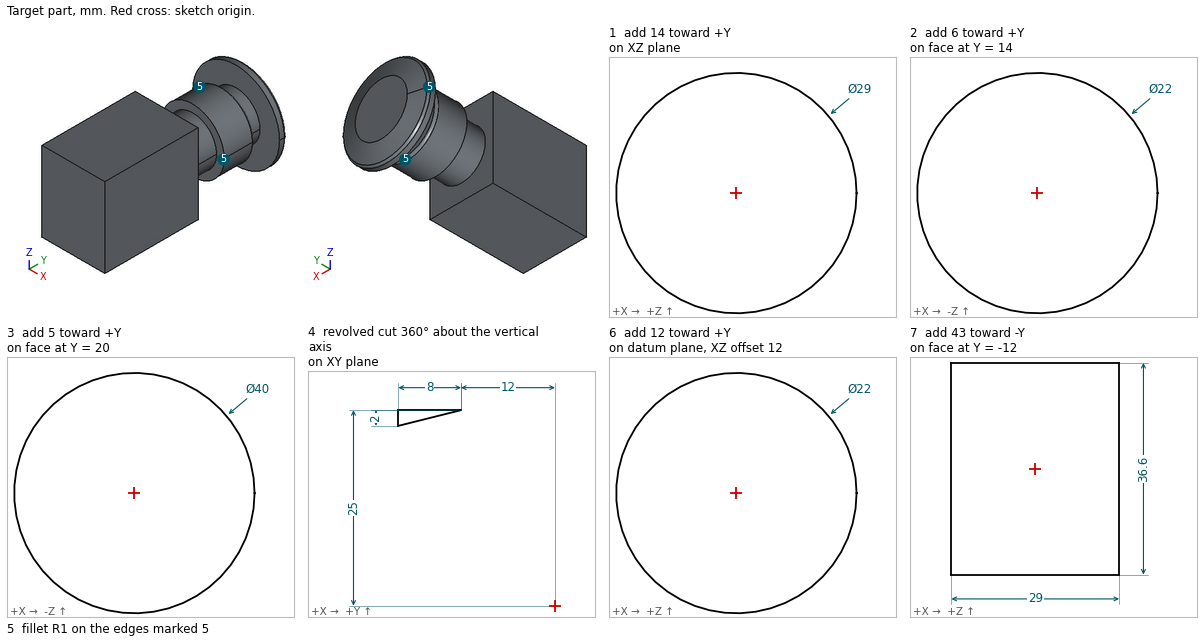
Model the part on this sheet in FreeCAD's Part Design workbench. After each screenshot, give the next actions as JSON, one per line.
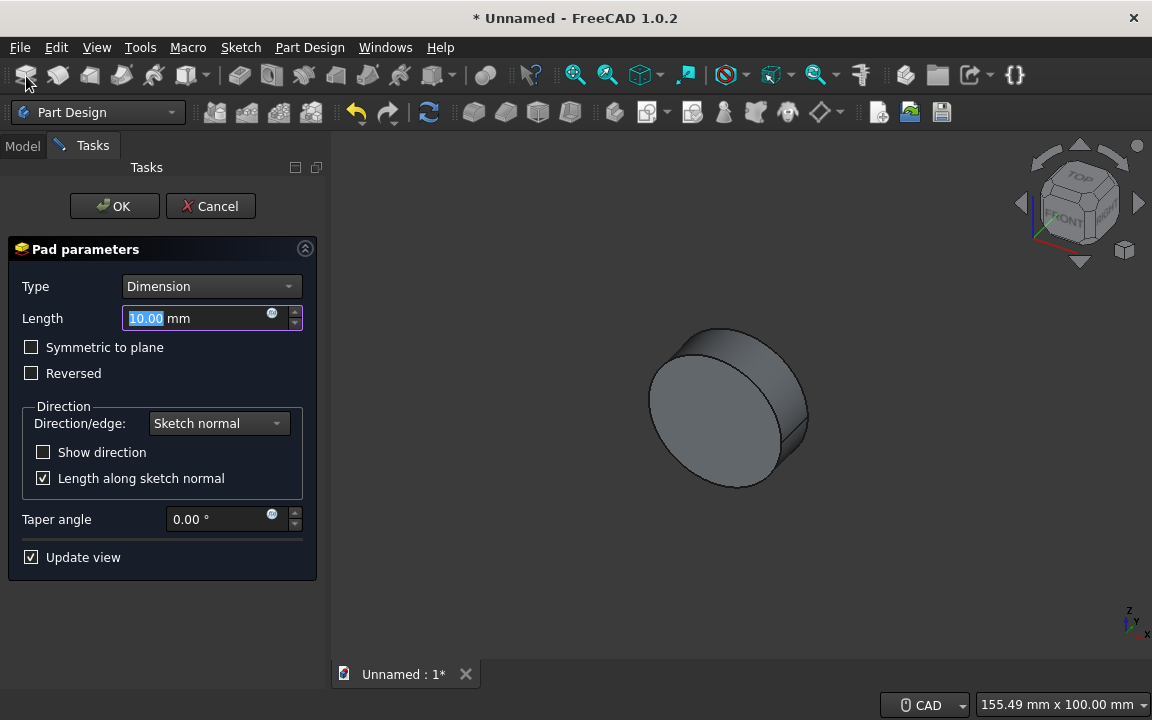
{"action": "type", "text": "14"}
{"action": "key", "text": "Tab"}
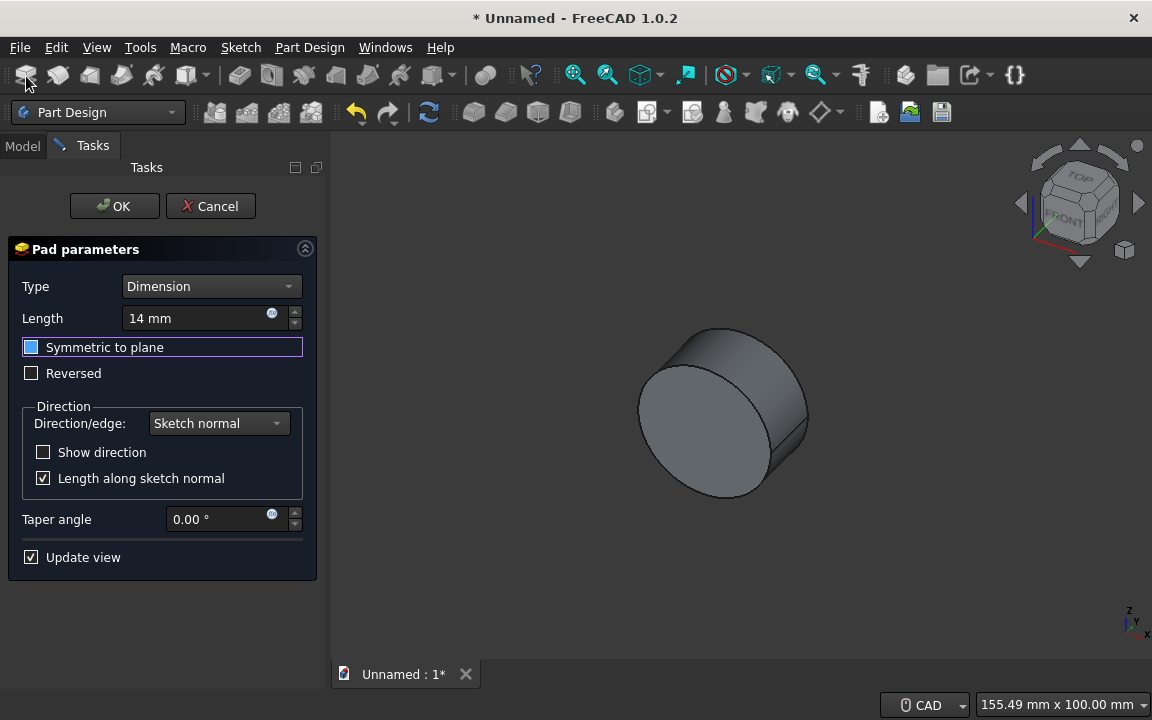
{"action": "left_click", "coordinate": [30, 373]}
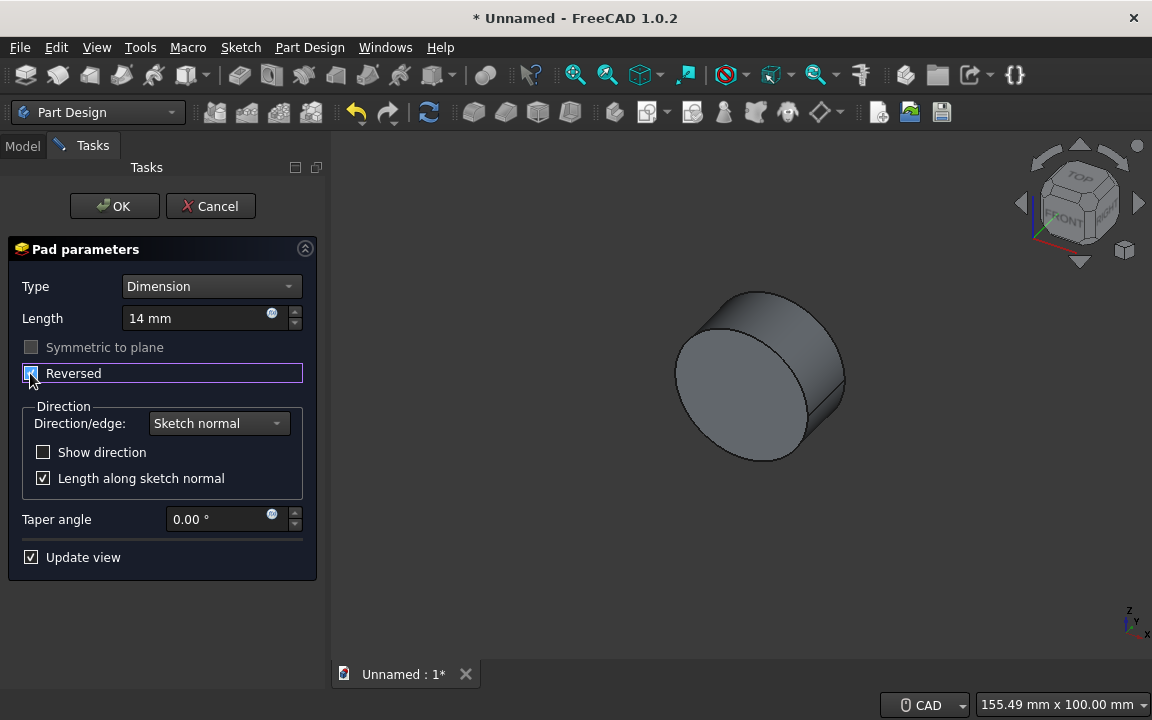
{"action": "left_click", "coordinate": [115, 206]}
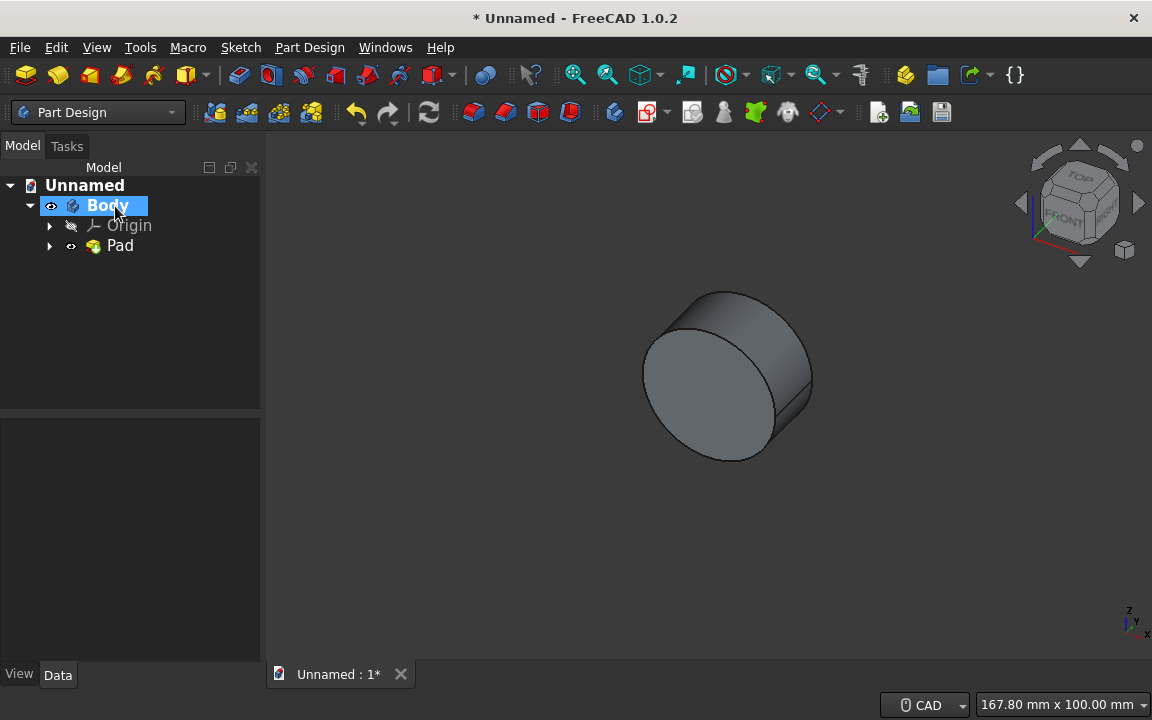
{"action": "left_click", "coordinate": [576, 76]}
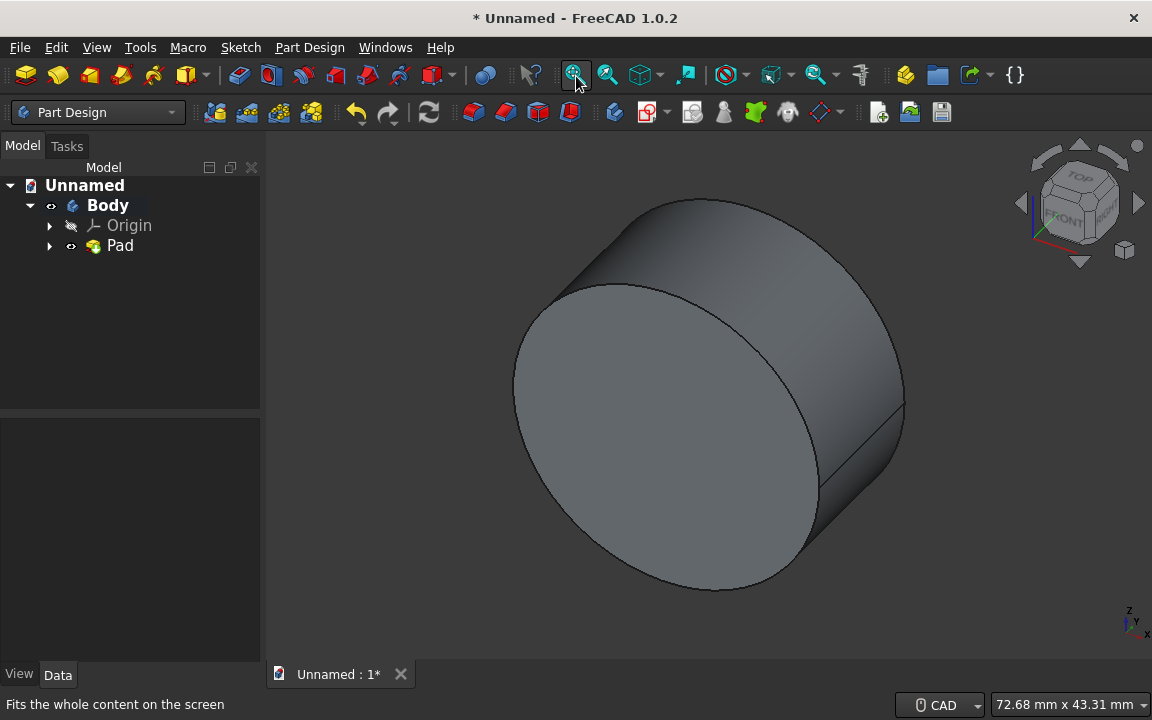
{"action": "key", "text": "4"}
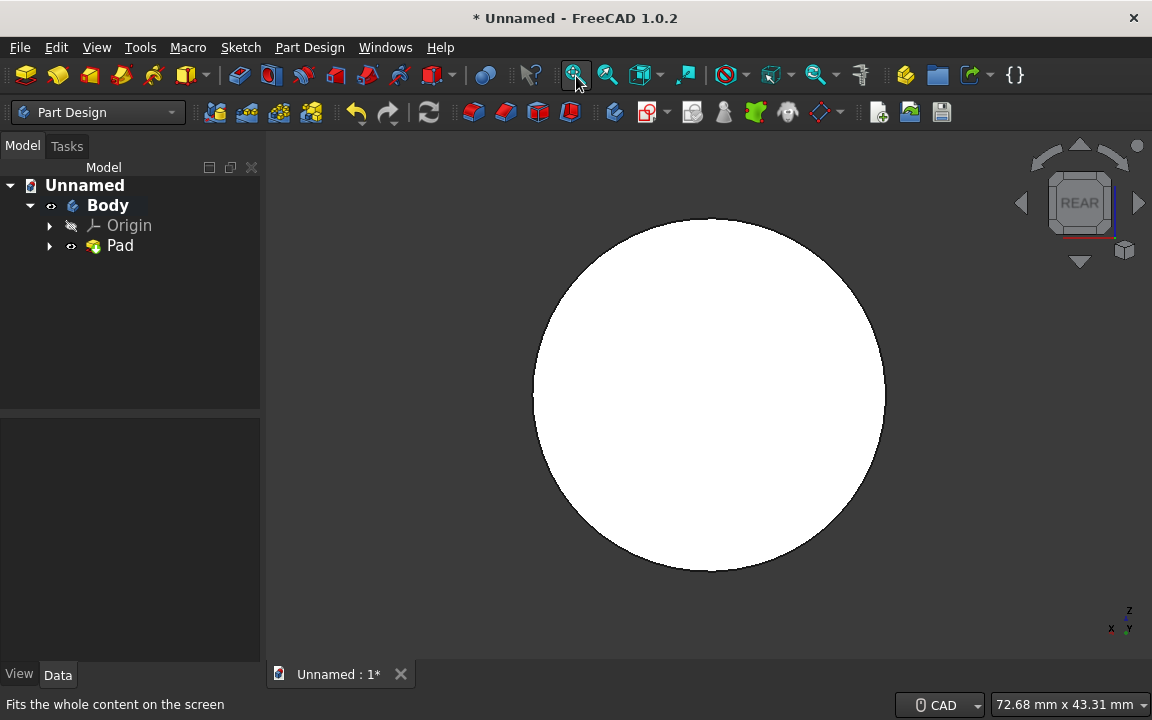
{"action": "left_click", "coordinate": [709, 394]}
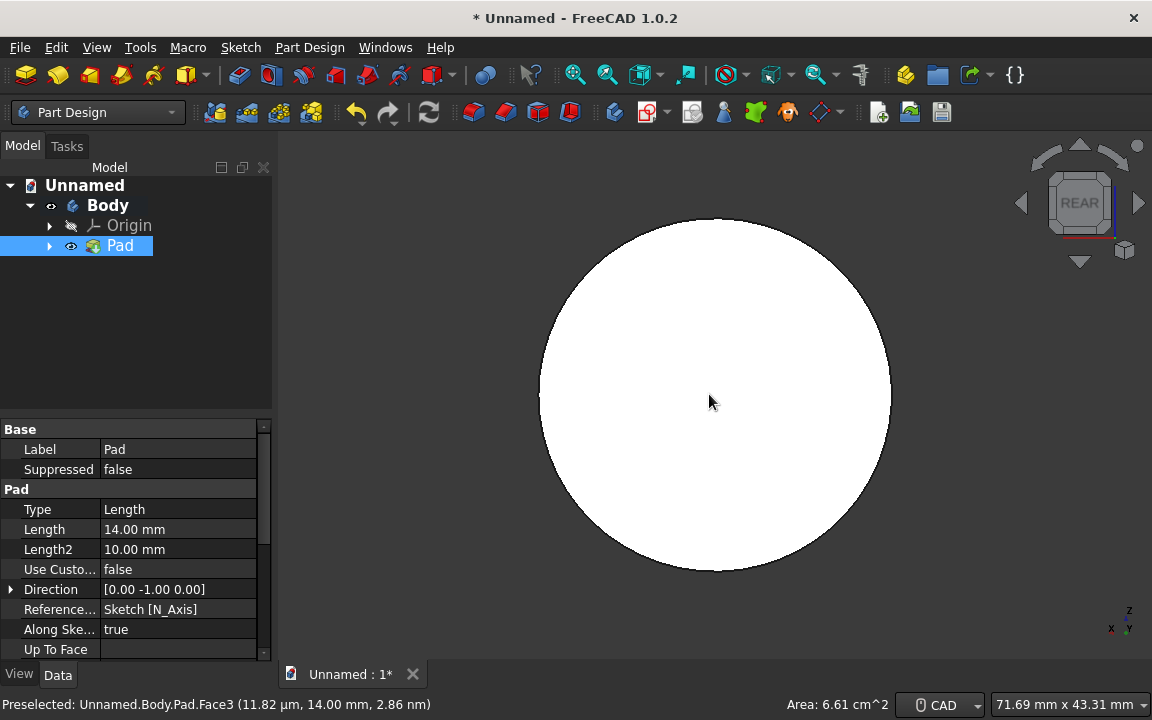
{"action": "left_click", "coordinate": [648, 112]}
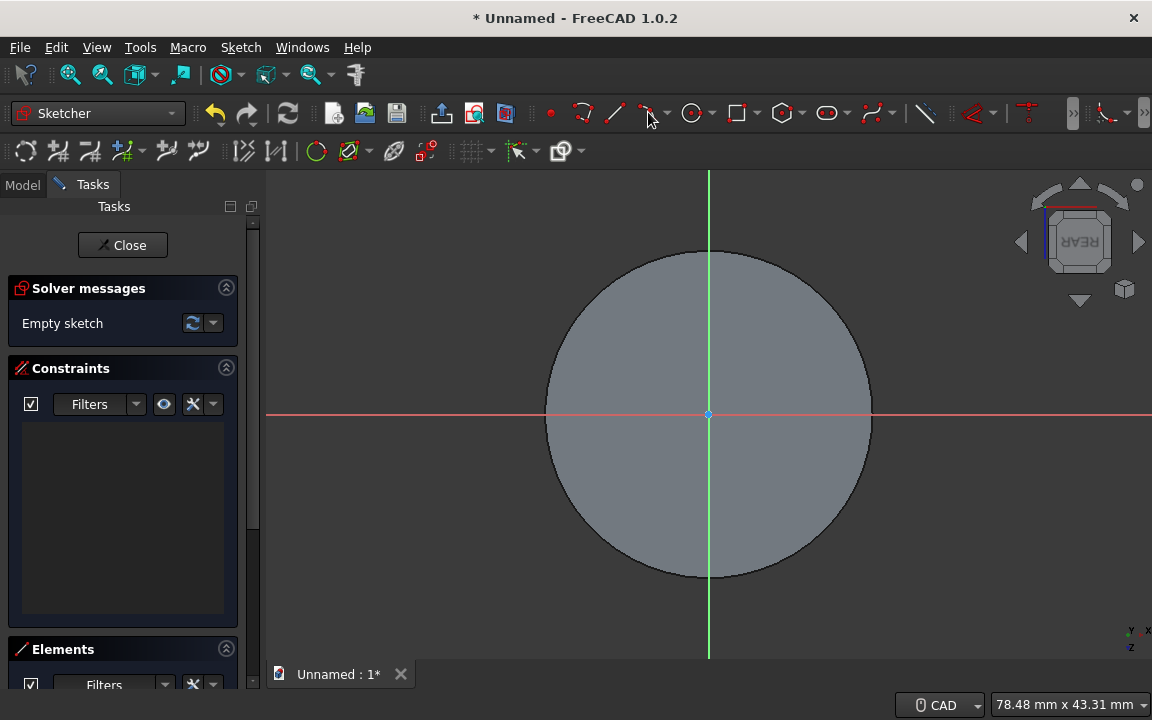
{"action": "key", "text": "g c"}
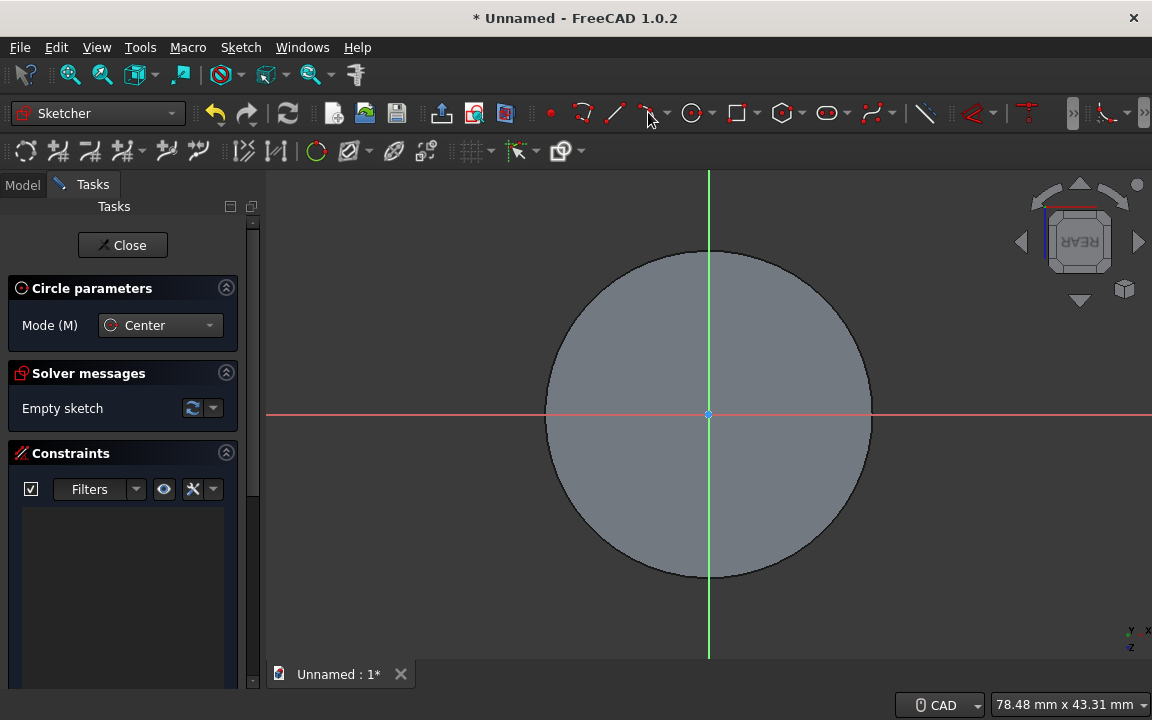
{"action": "left_click", "coordinate": [709, 414]}
{"action": "left_click", "coordinate": [797, 327]}
{"action": "key", "text": "Escape"}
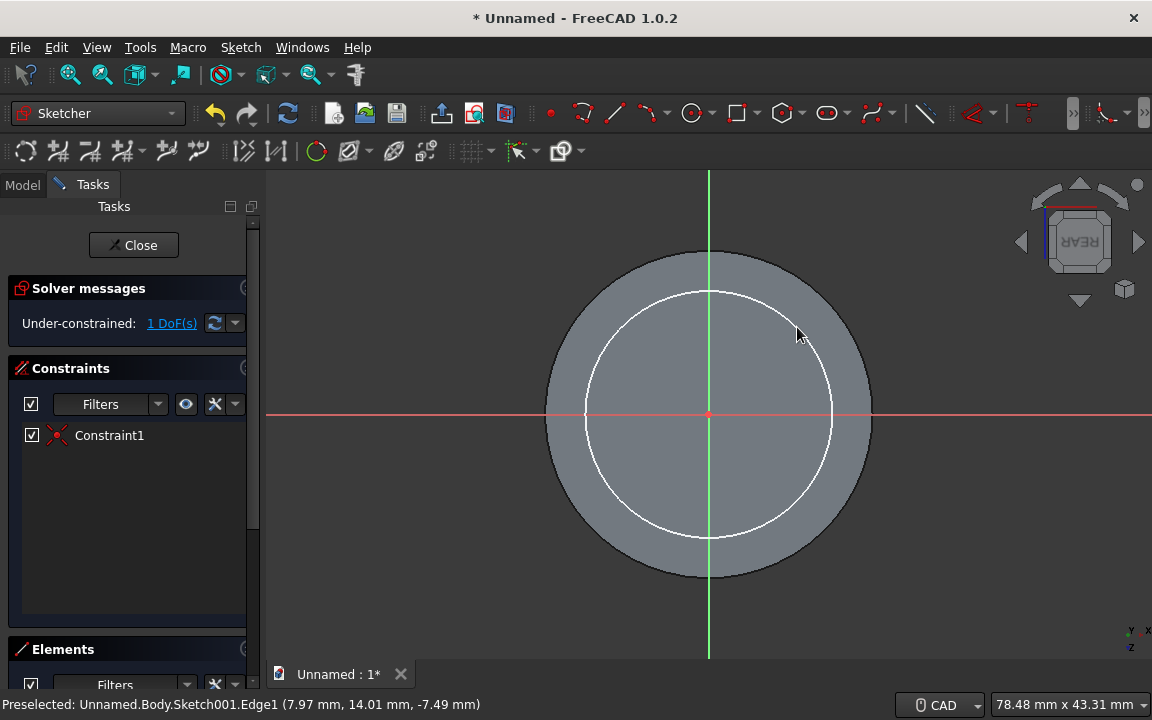
{"action": "left_click", "coordinate": [796, 327]}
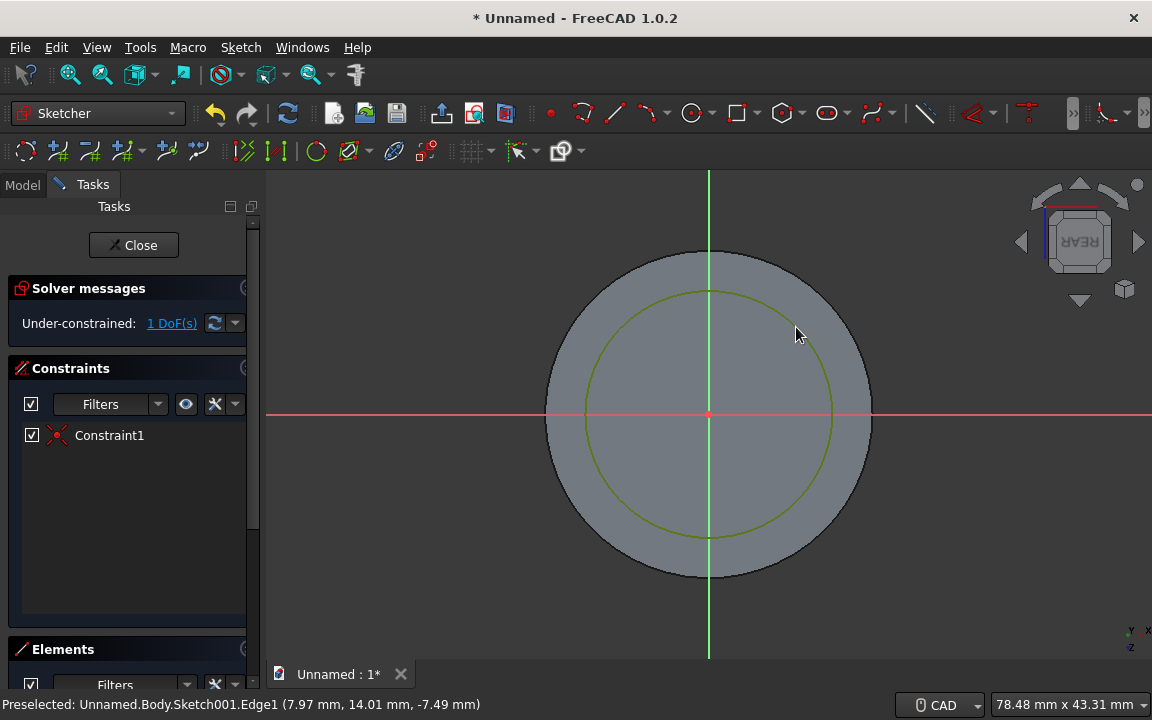
{"action": "key", "text": "k o"}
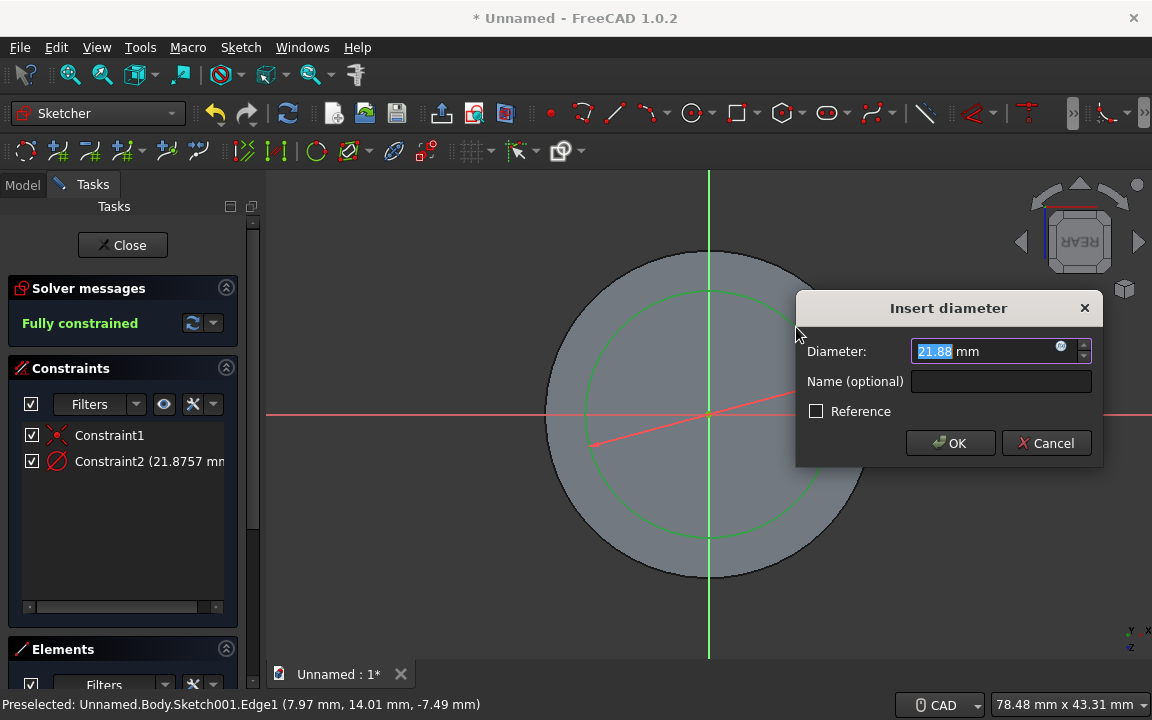
{"action": "type", "text": "22"}
{"action": "key", "text": "Return"}